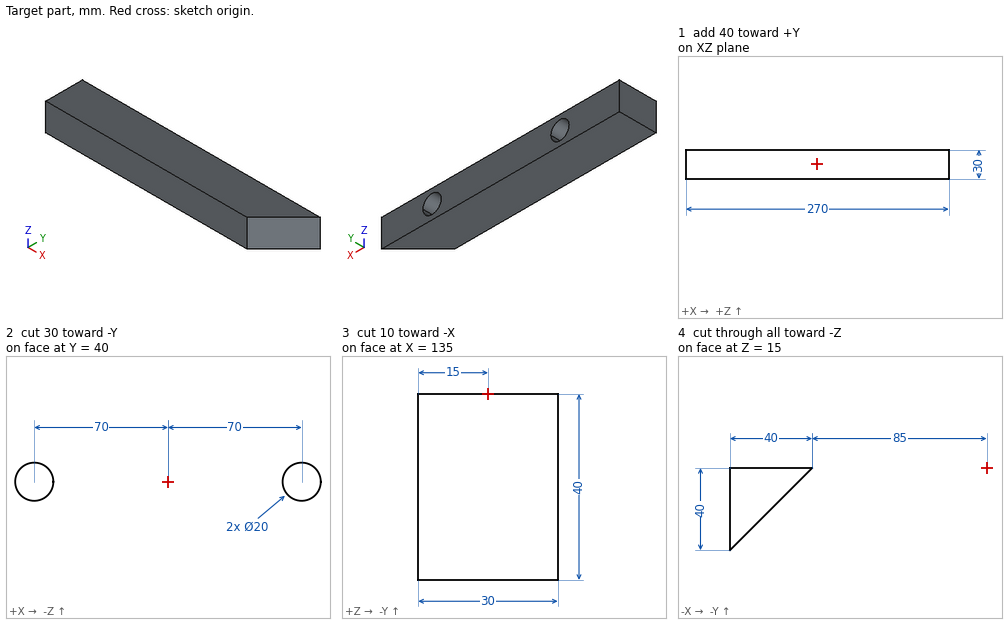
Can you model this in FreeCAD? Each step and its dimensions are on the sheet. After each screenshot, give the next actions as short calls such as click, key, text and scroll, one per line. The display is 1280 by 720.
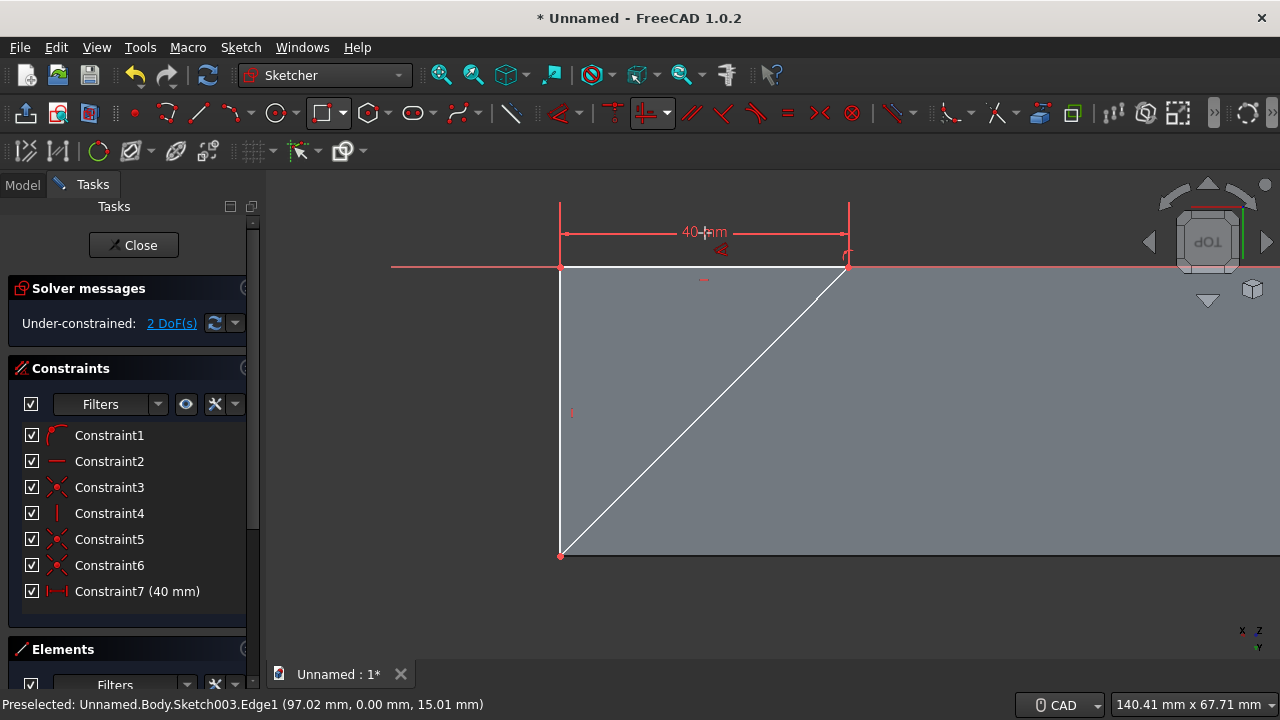
click(560, 354)
click(526, 412)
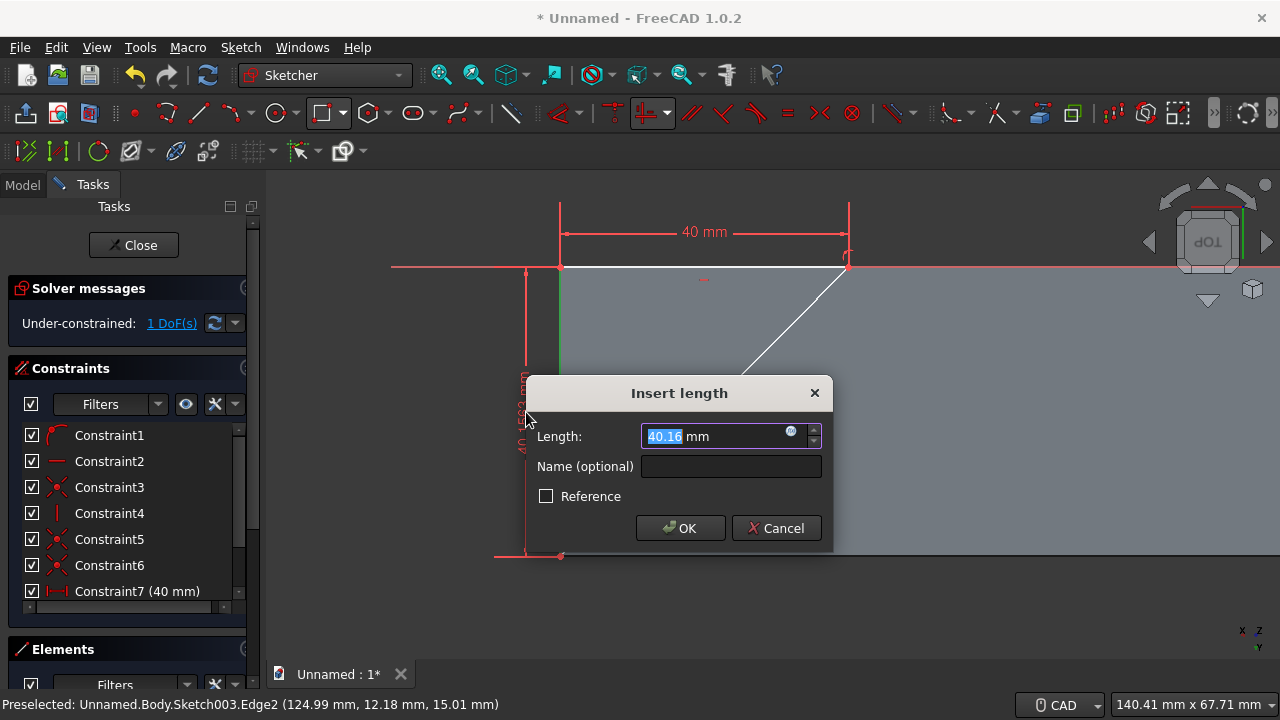
text(40)
key(Return)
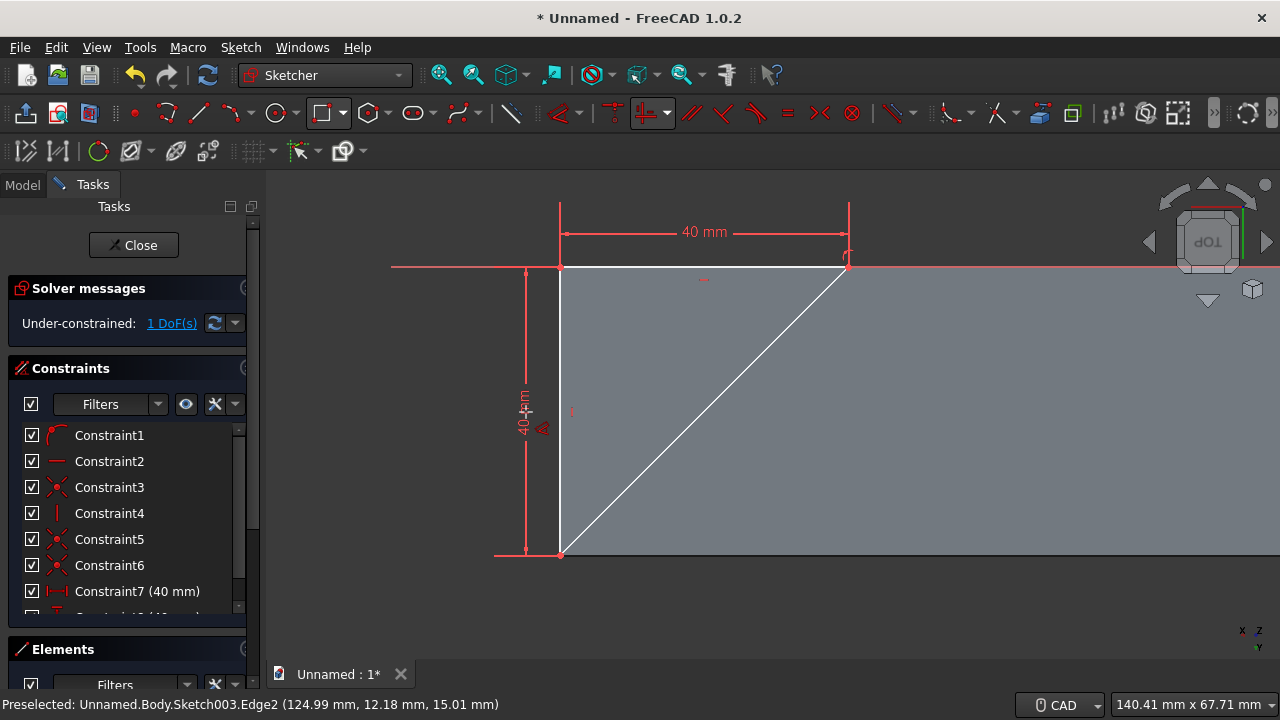
click(849, 267)
click(982, 233)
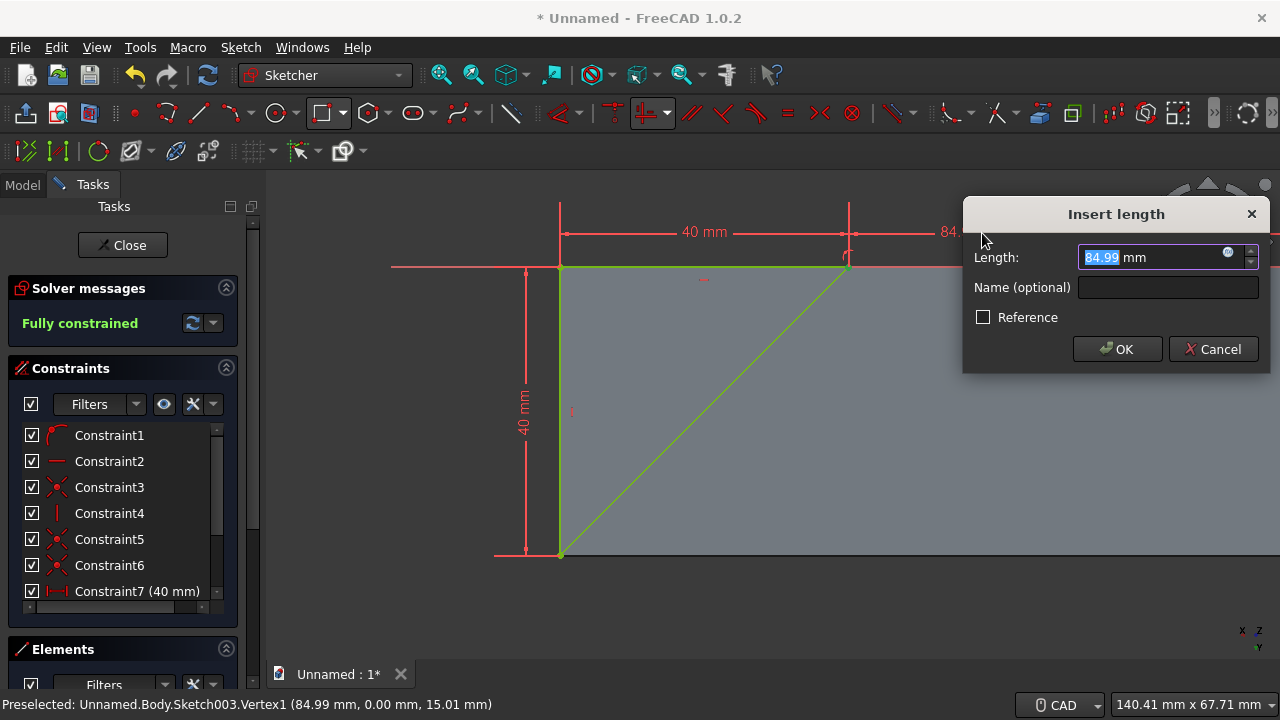
text(85)
key(Return)
key(Escape)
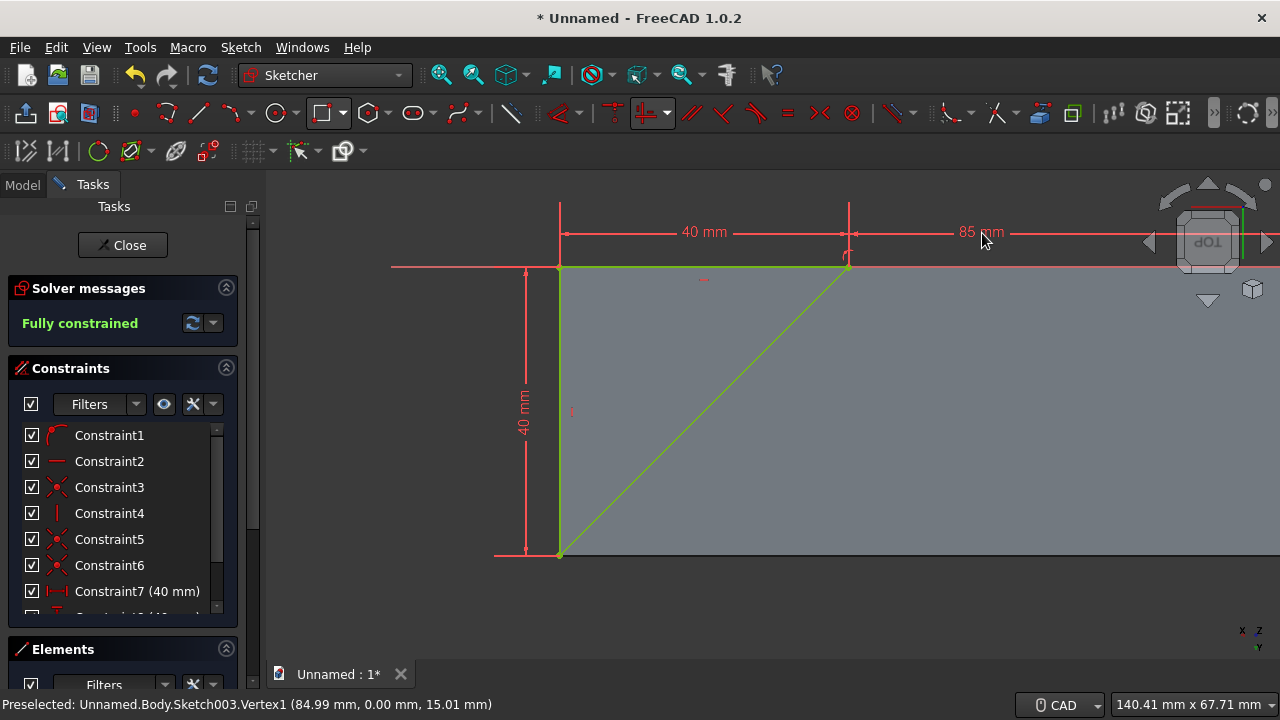
click(123, 245)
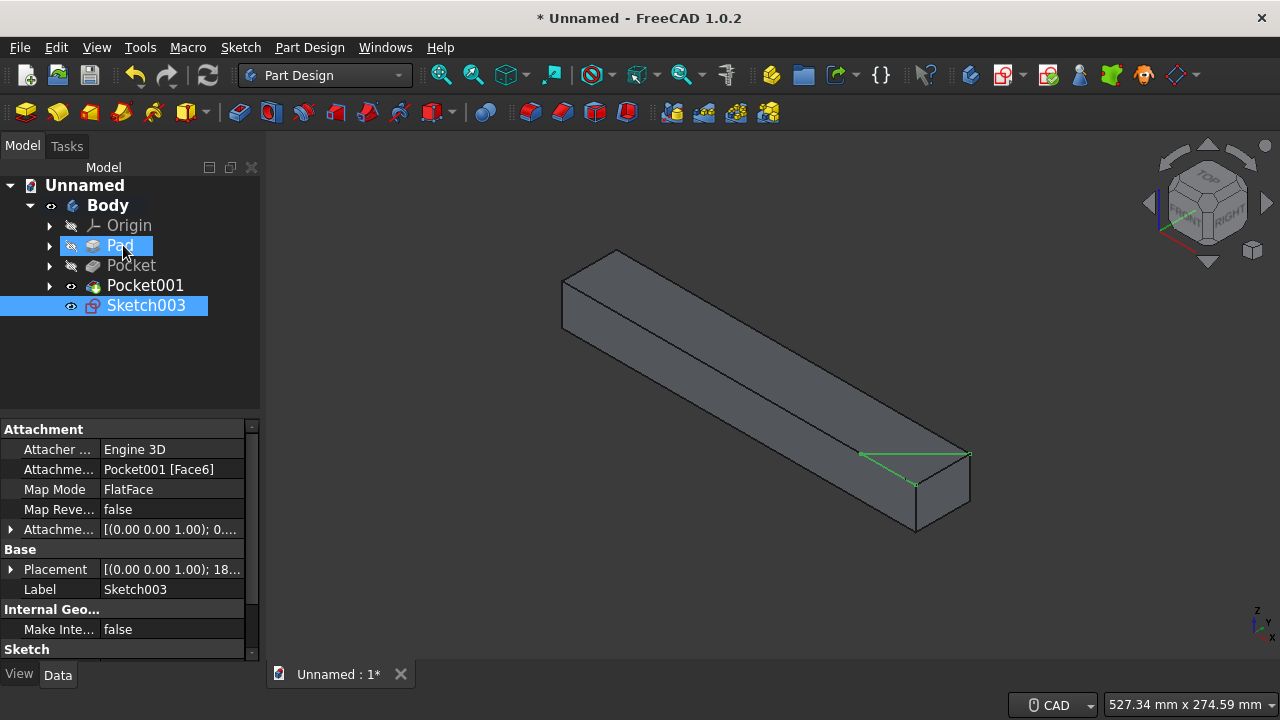
click(240, 112)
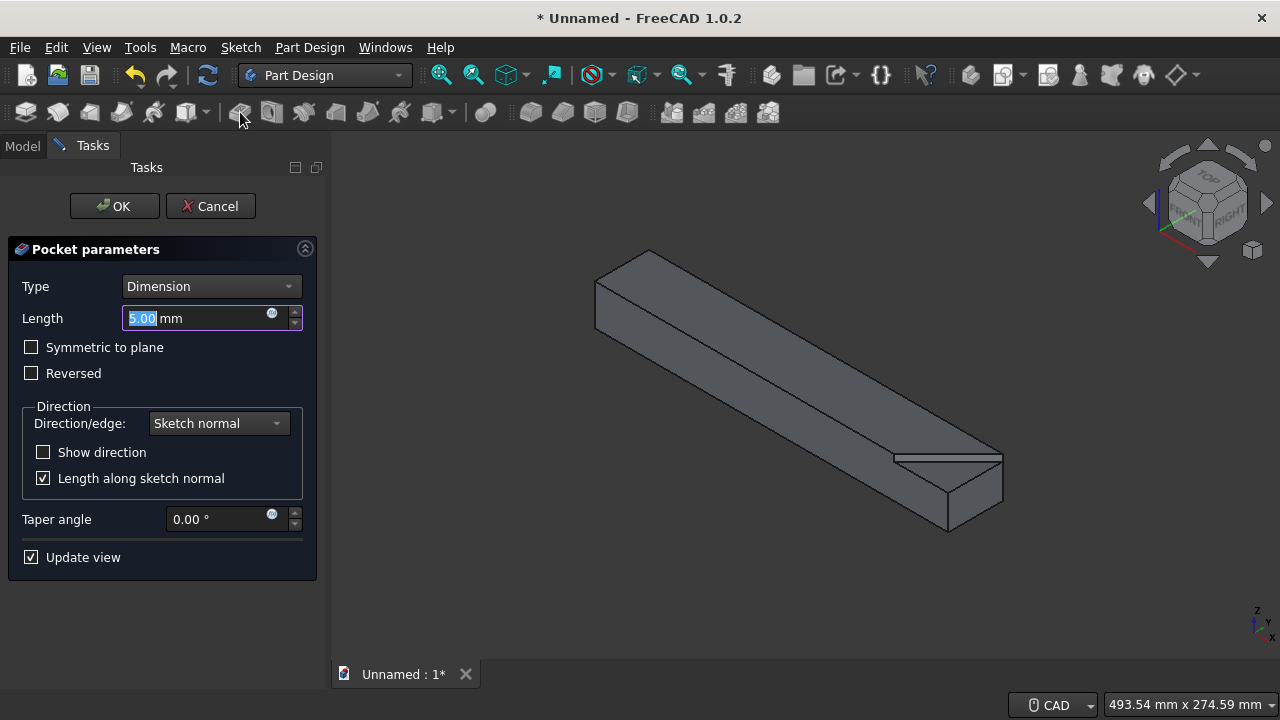
click(212, 286)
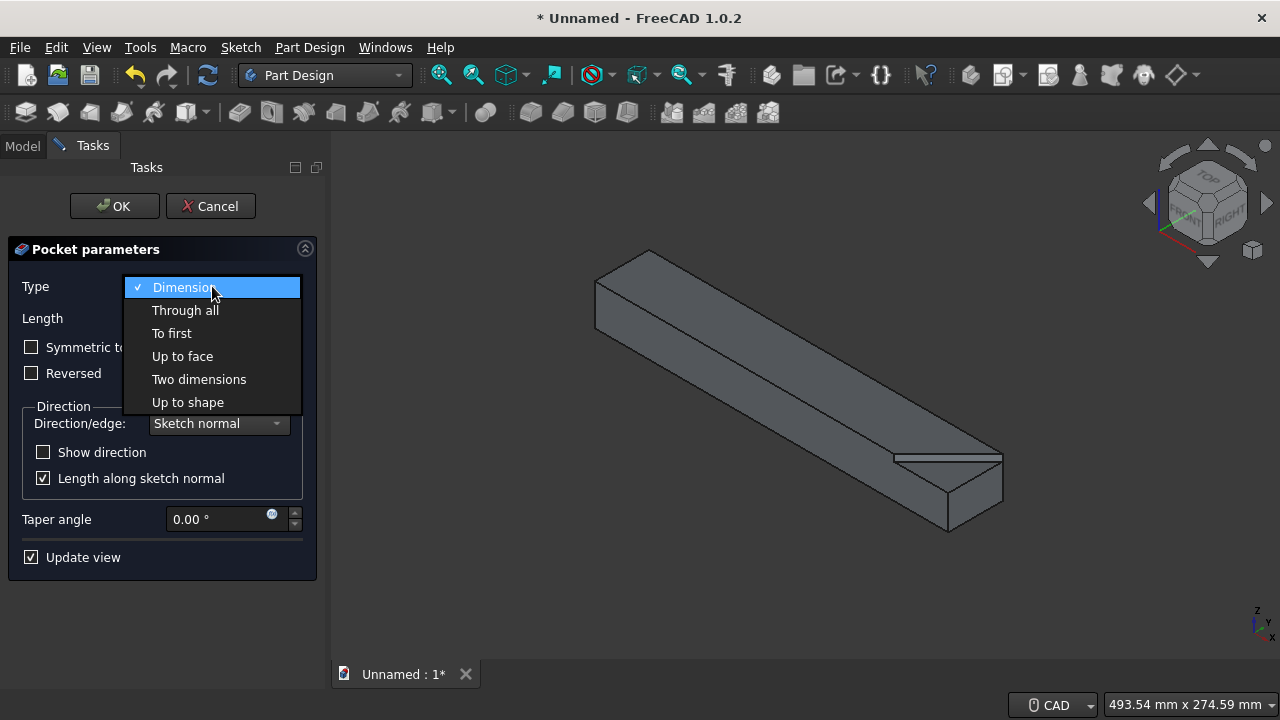
click(212, 310)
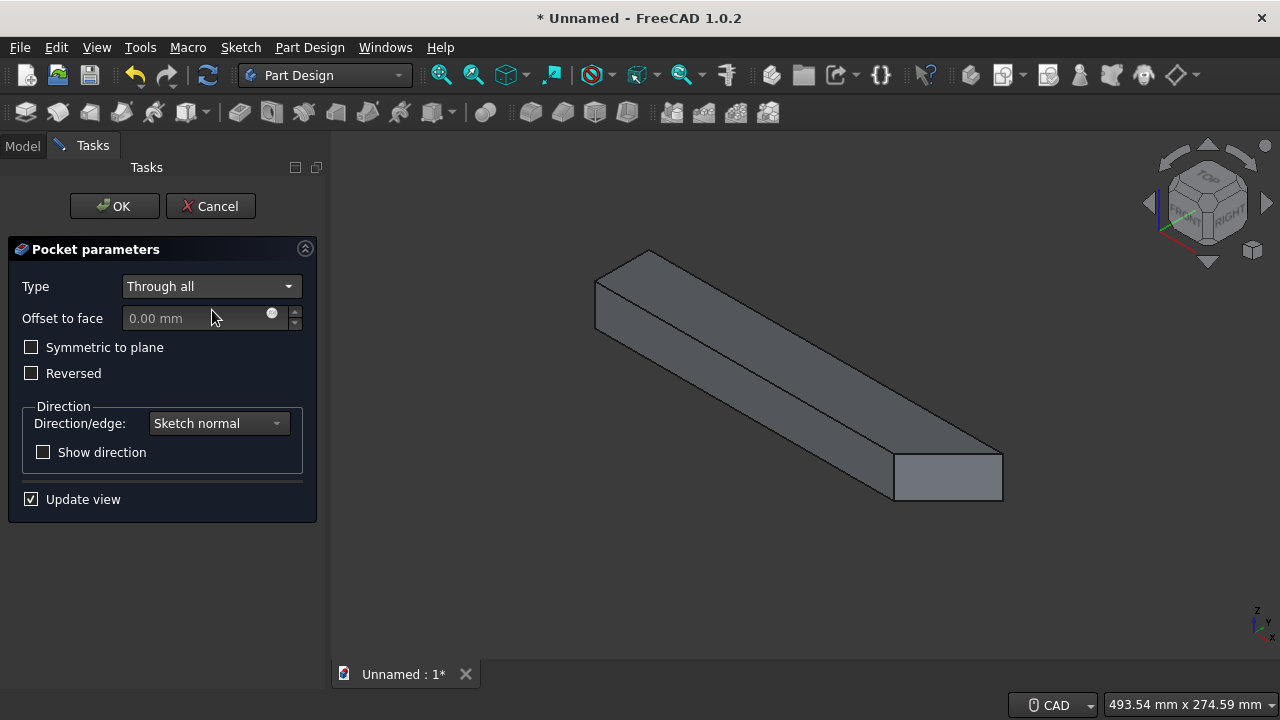
click(115, 206)